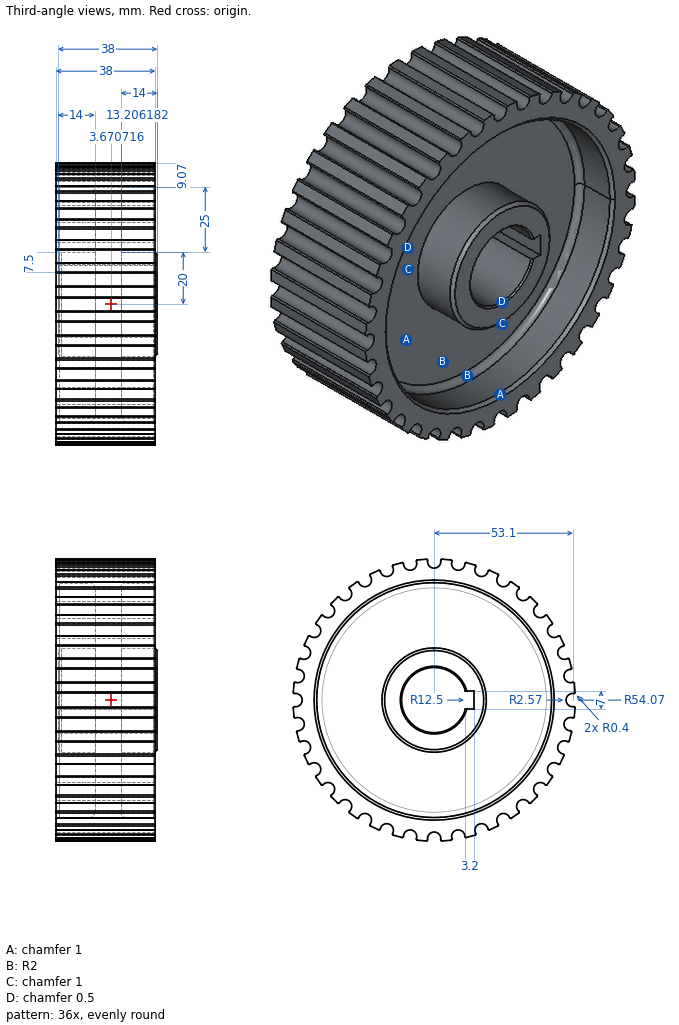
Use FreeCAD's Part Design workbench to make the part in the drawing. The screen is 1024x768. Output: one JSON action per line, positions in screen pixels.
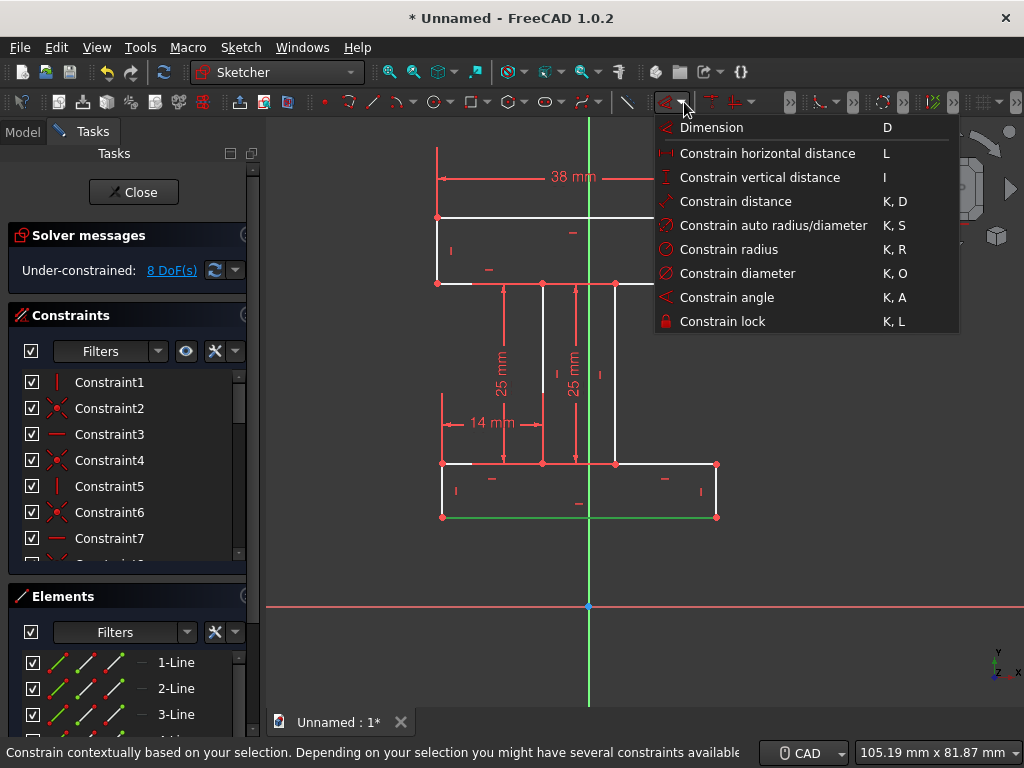
{"action": "left_click", "coordinate": [807, 153]}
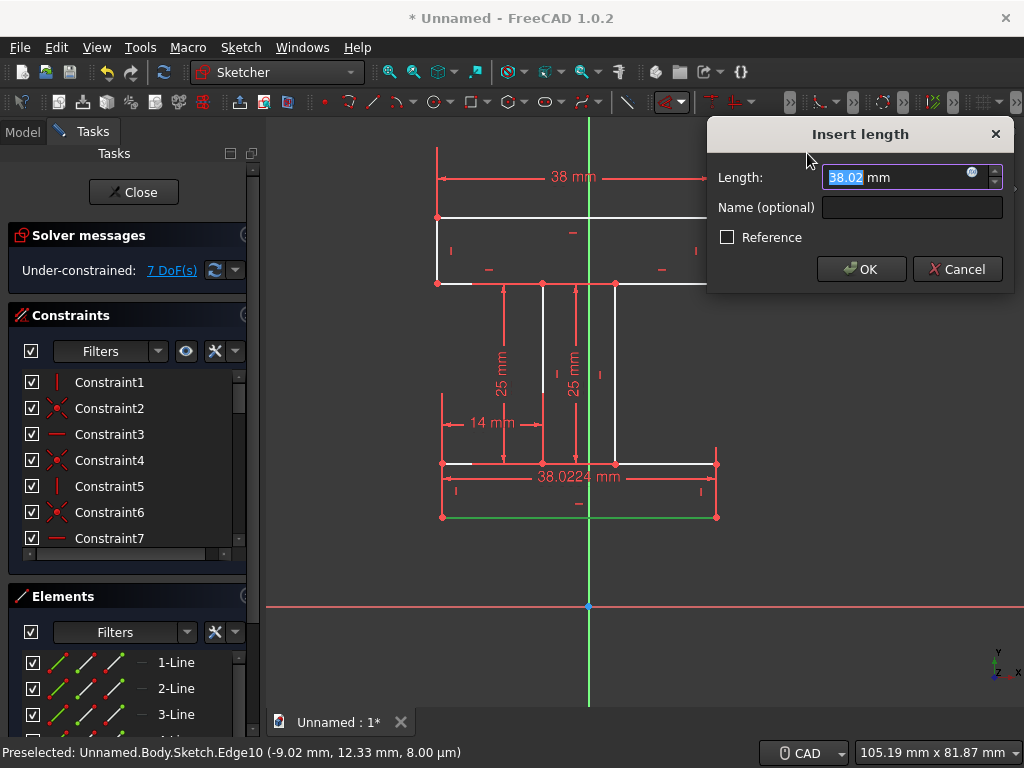
{"action": "type", "text": "38"}
{"action": "key", "text": "Return"}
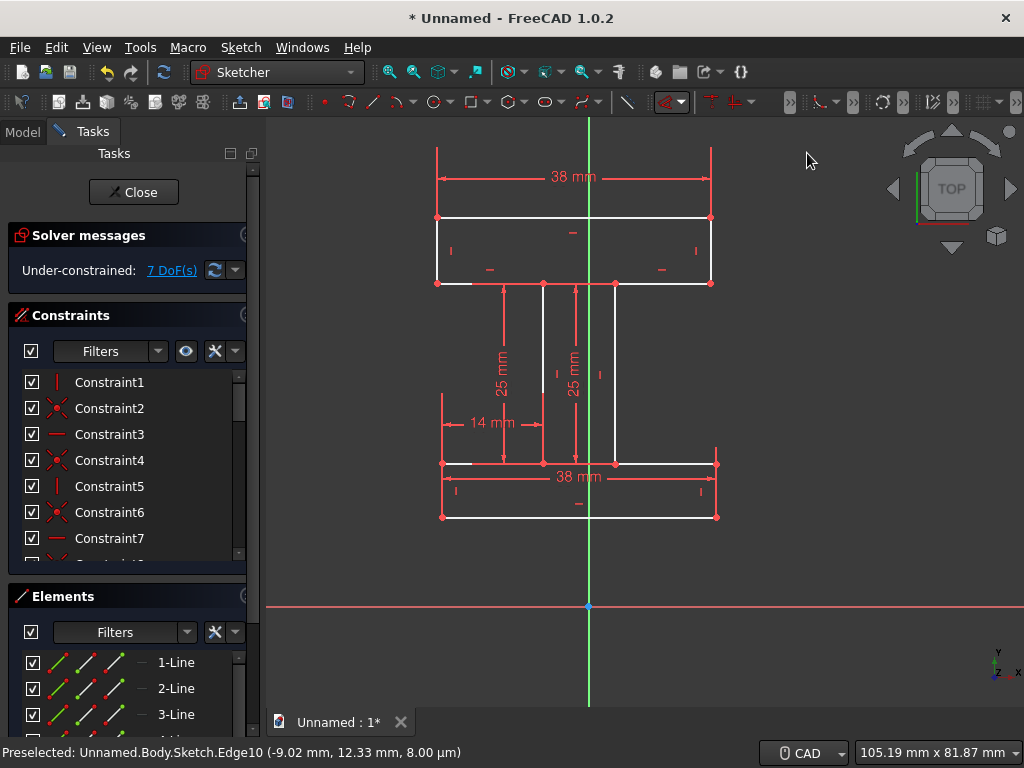
{"action": "left_click", "coordinate": [686, 464]}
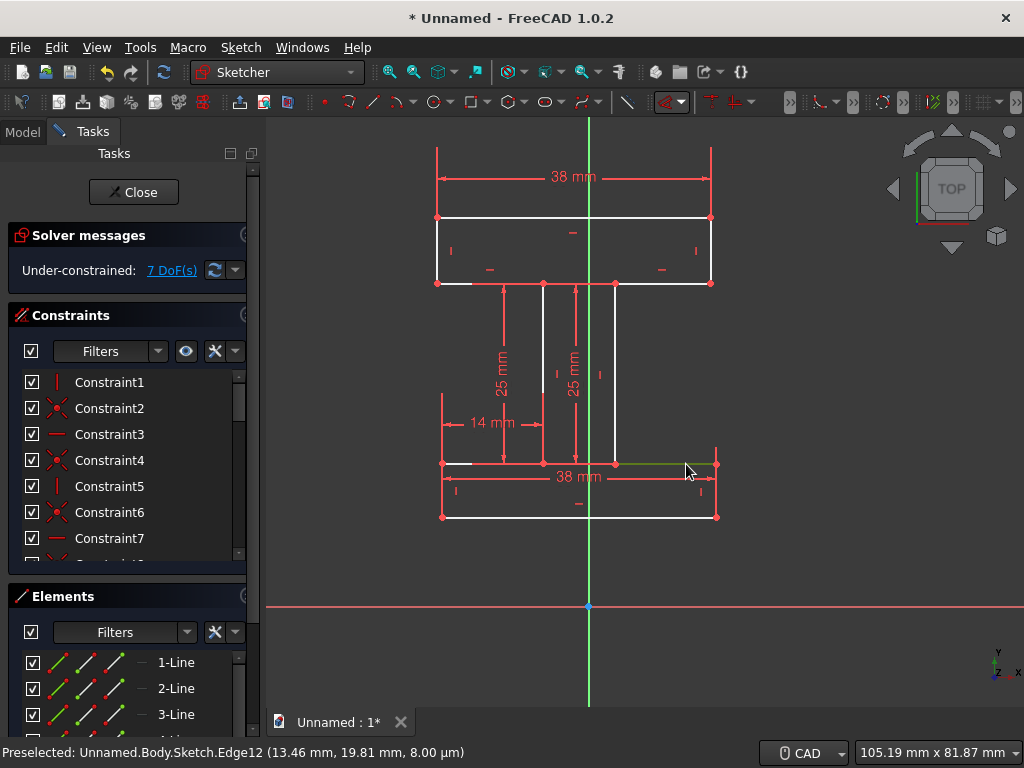
{"action": "key", "text": "l"}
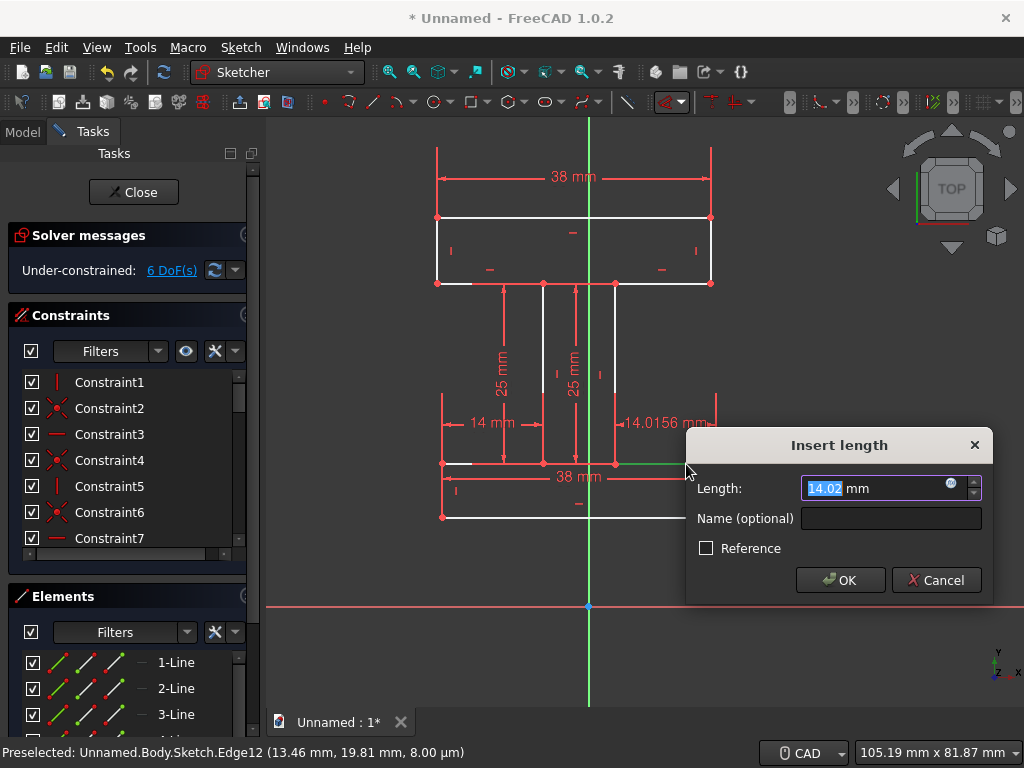
{"action": "type", "text": "14"}
{"action": "key", "text": "Return"}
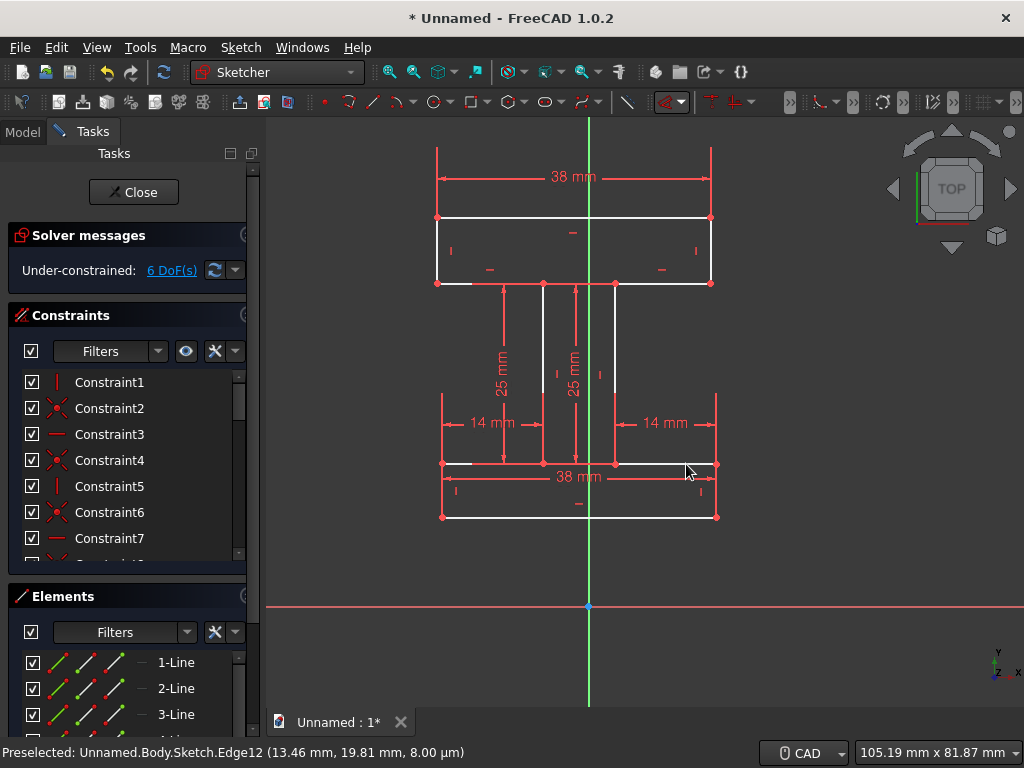
{"action": "left_click", "coordinate": [442, 480]}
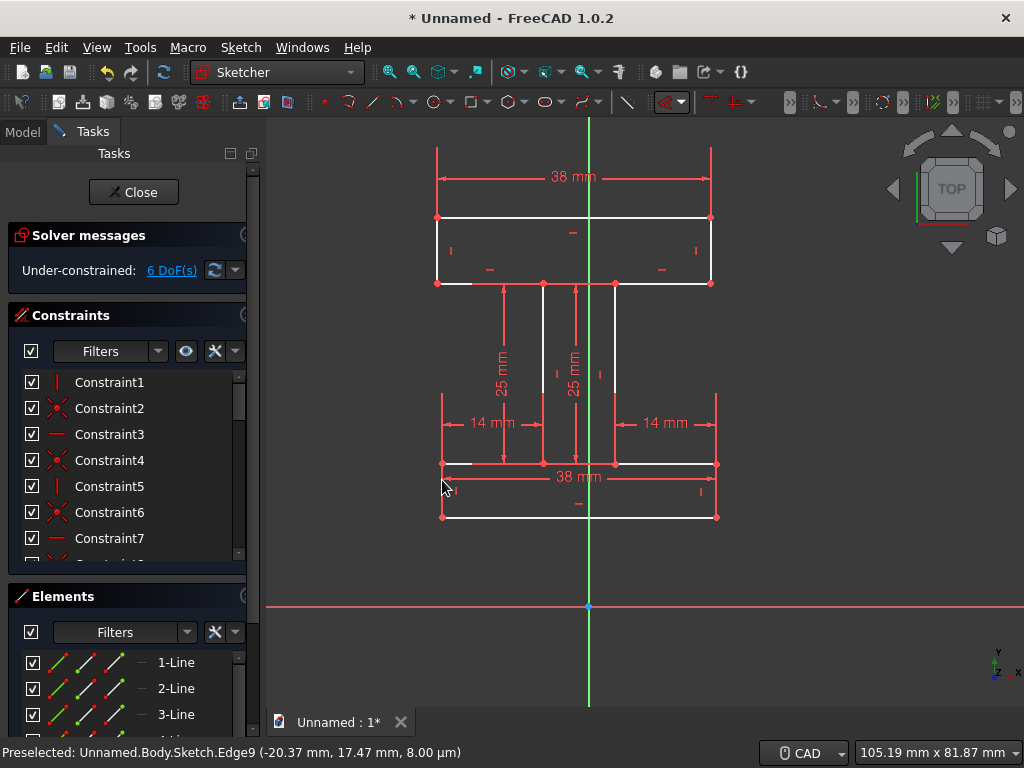
{"action": "key", "text": "i"}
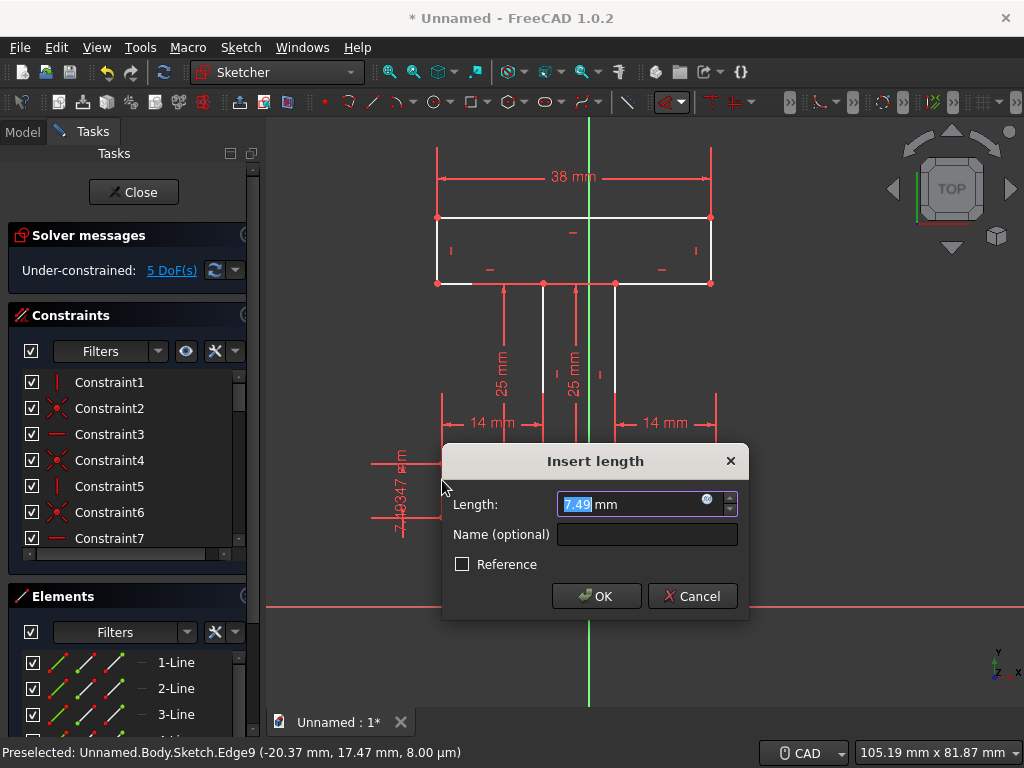
{"action": "type", "text": "7.5"}
{"action": "key", "text": "Return"}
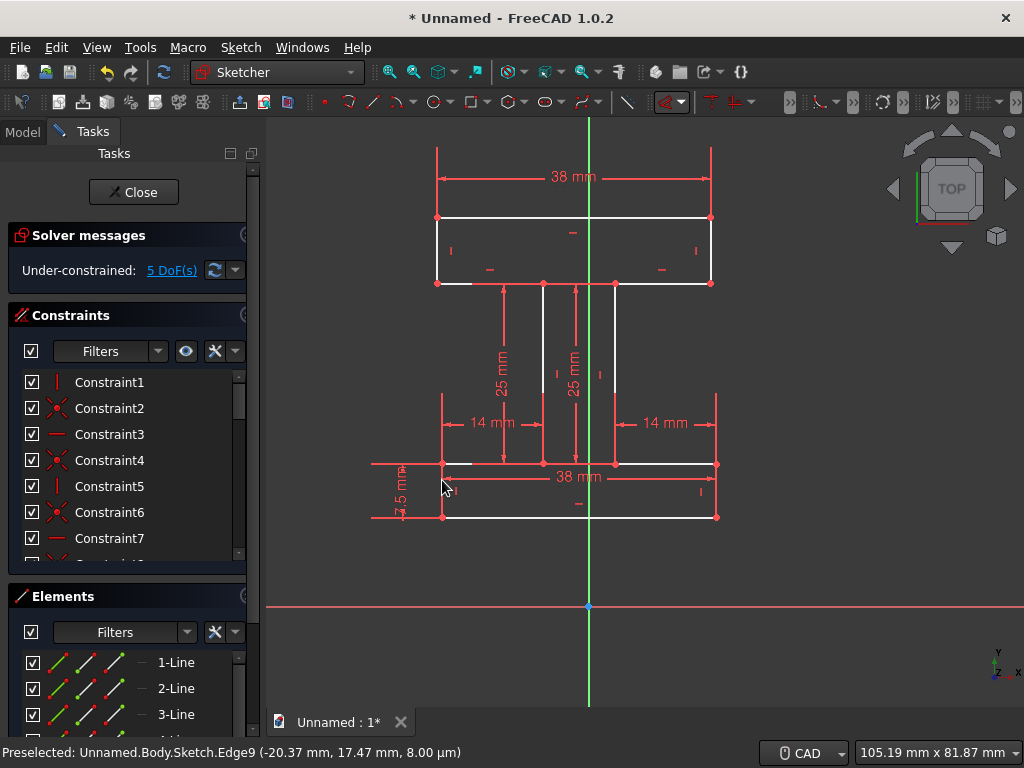
{"action": "left_click", "coordinate": [716, 502]}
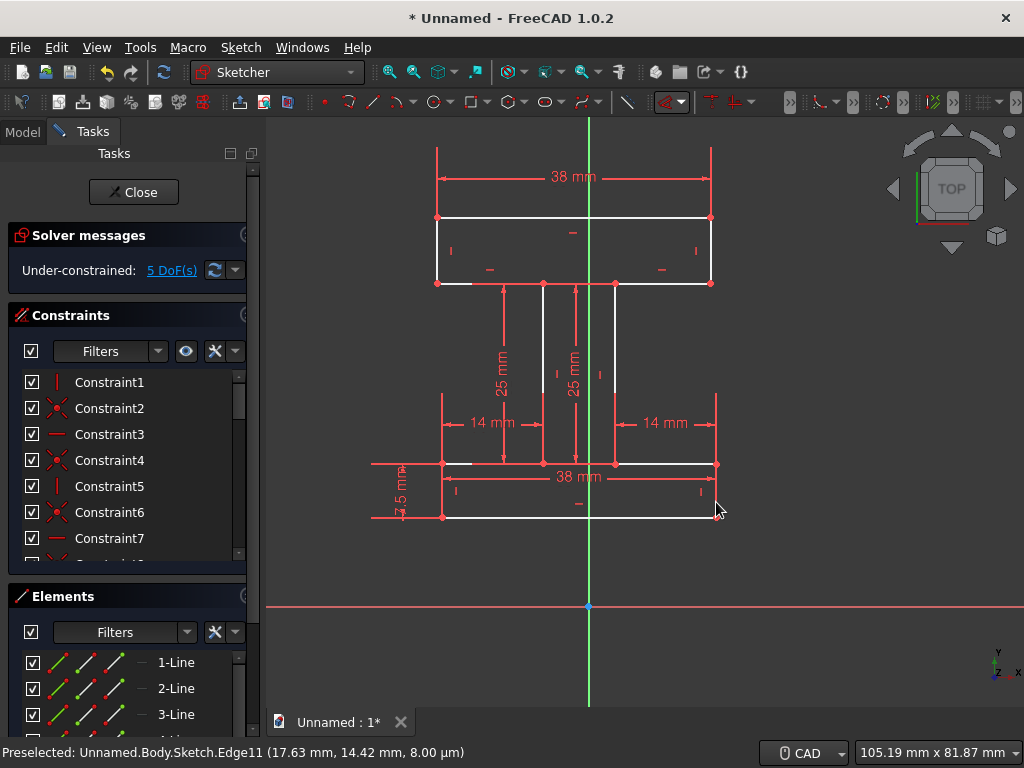
{"action": "key", "text": "i"}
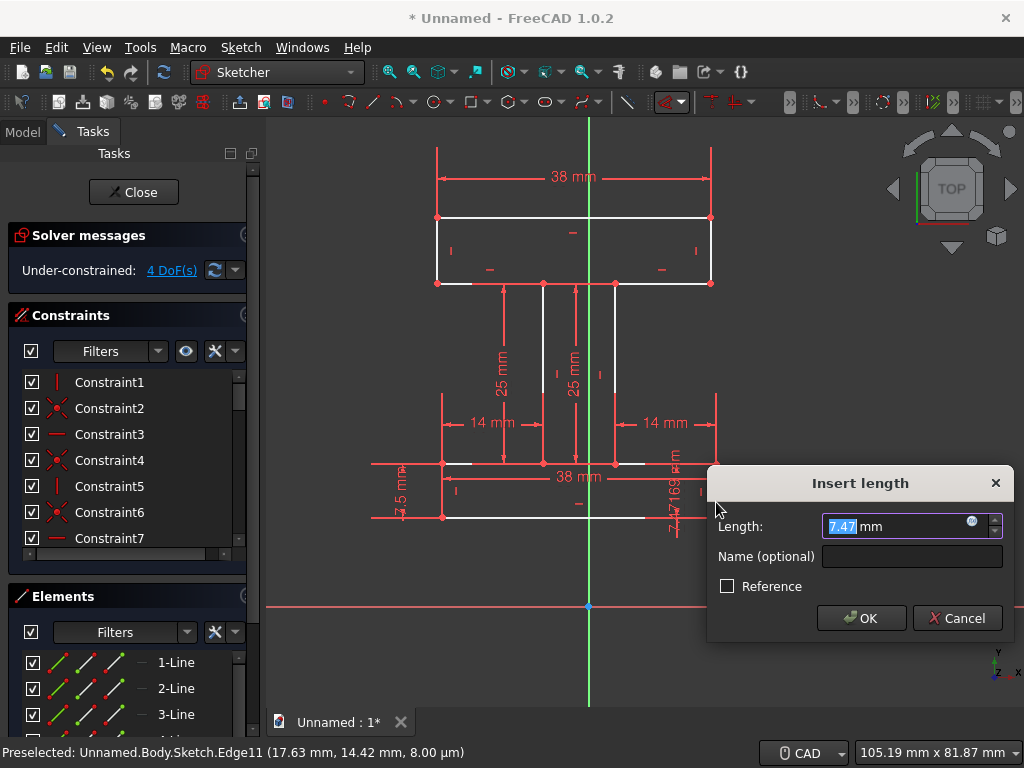
{"action": "type", "text": "7.5"}
{"action": "key", "text": "Return"}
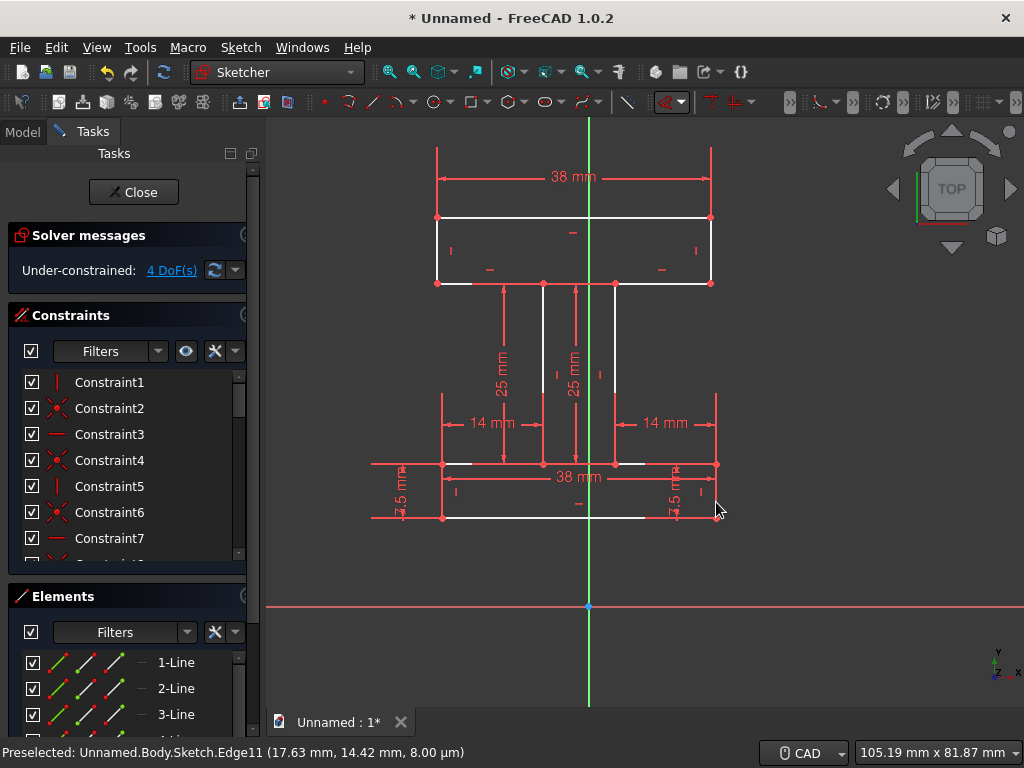
{"action": "left_click", "coordinate": [615, 464]}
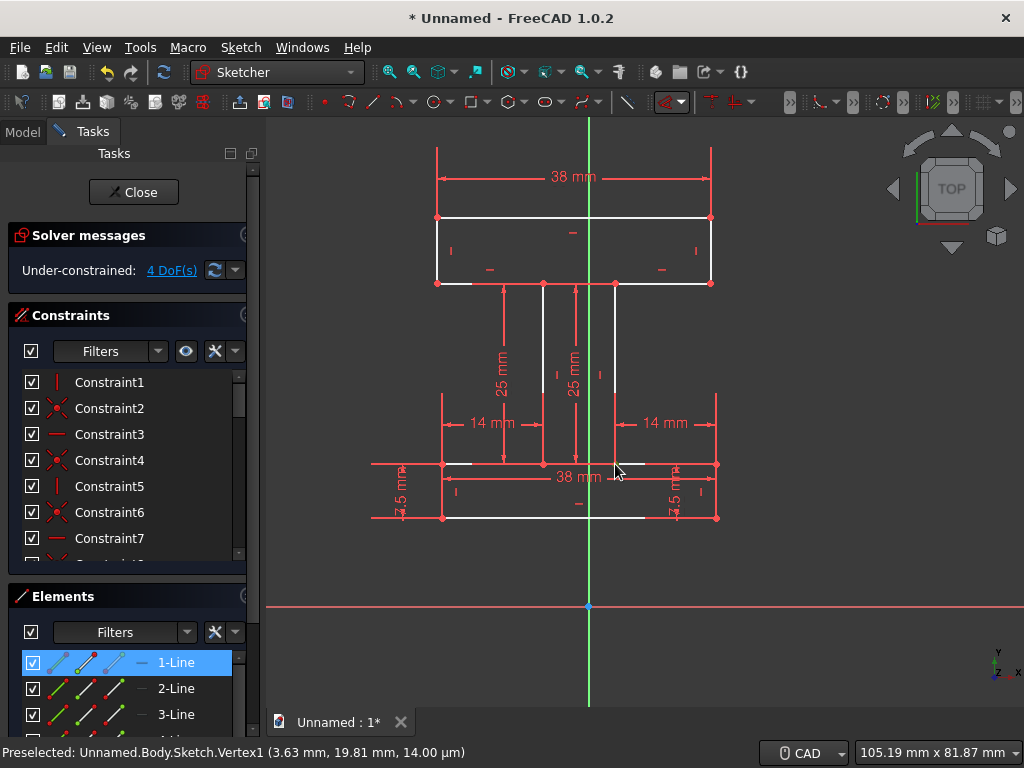
{"action": "left_click", "coordinate": [684, 102]}